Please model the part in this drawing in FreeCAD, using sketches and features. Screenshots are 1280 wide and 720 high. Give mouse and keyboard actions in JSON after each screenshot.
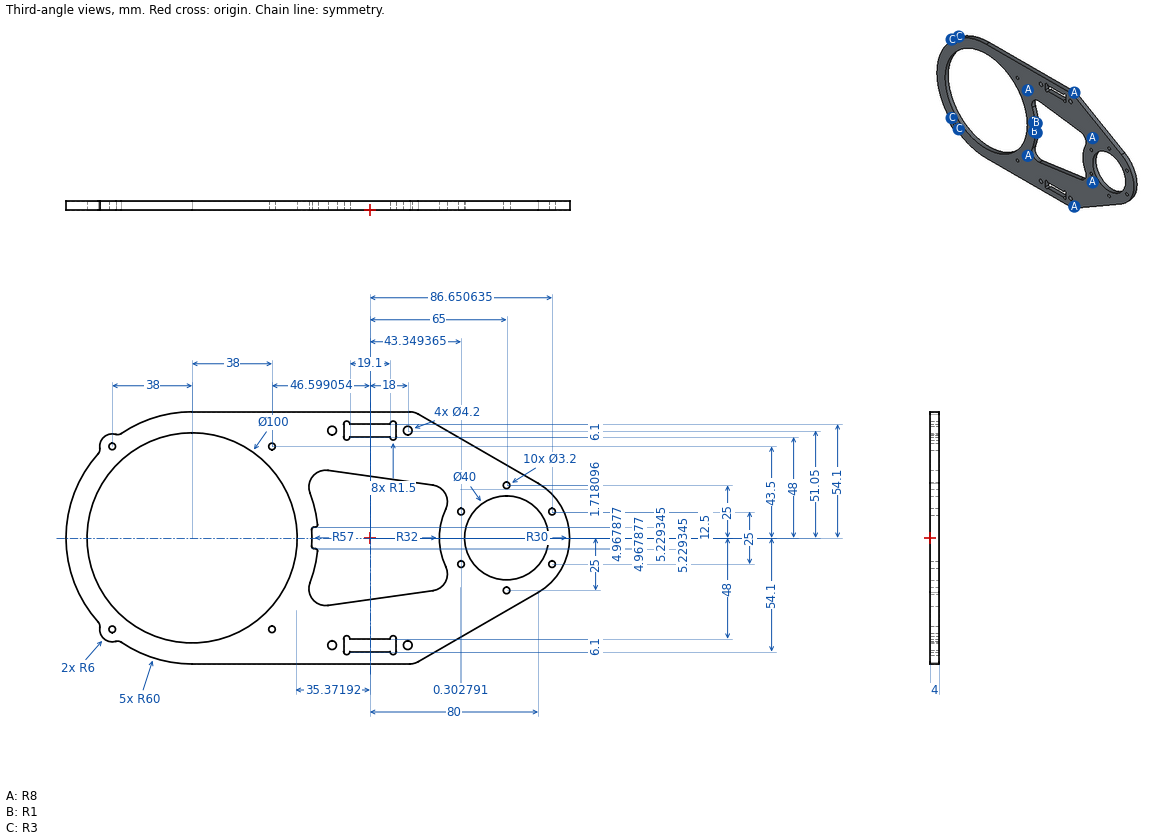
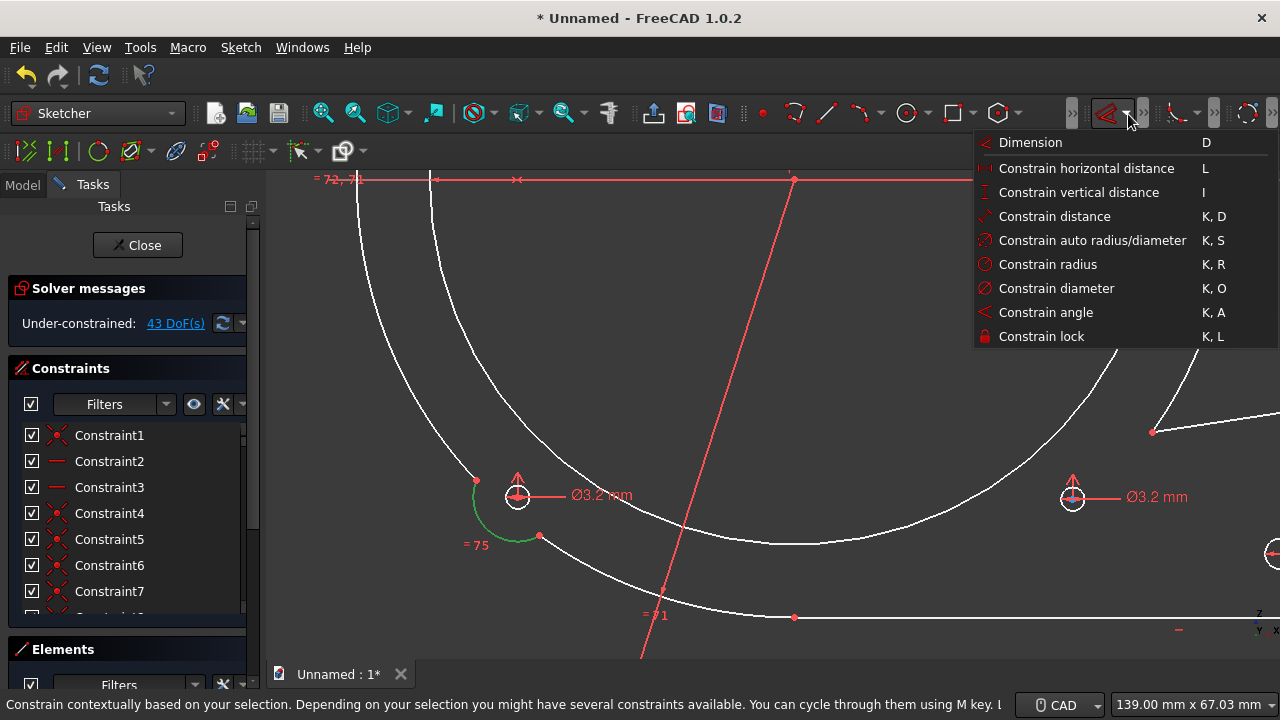
{"action": "left_click", "coordinate": [1126, 264]}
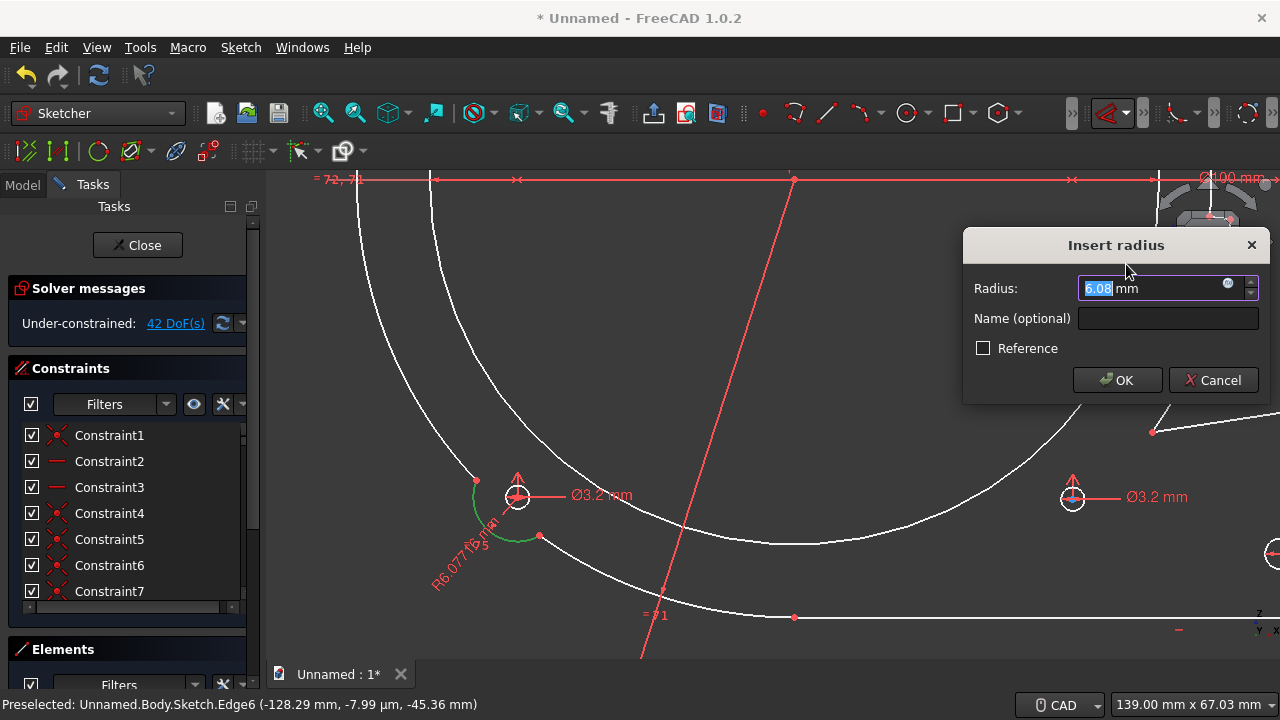
{"action": "type", "text": "6"}
{"action": "key", "text": "Return"}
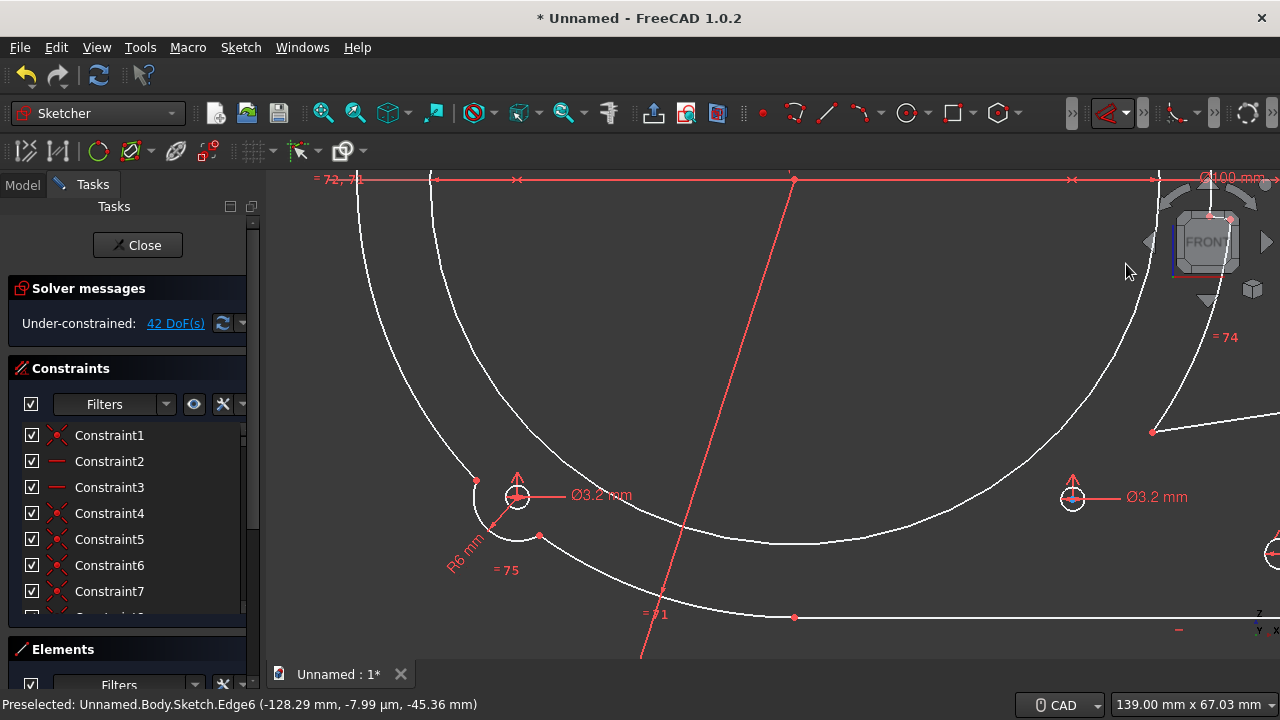
{"action": "scroll", "coordinate": [478, 516], "scroll_direction": "down", "scroll_amount": 6}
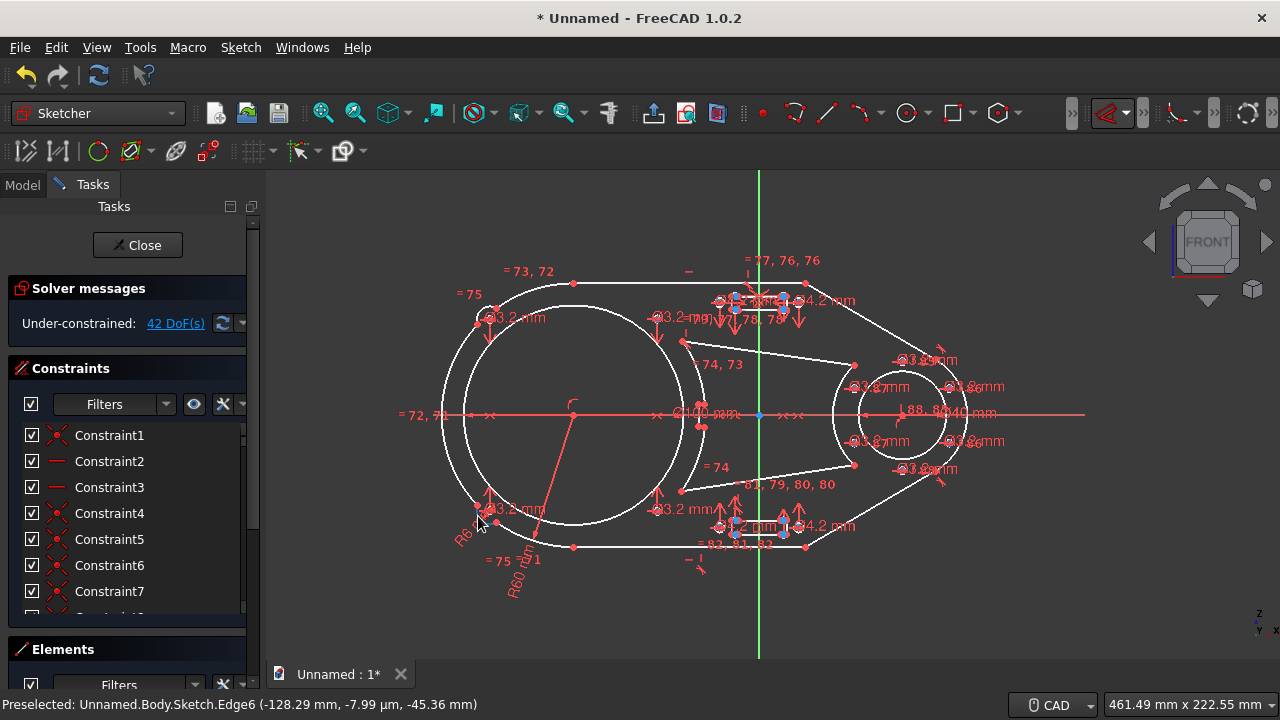
{"action": "scroll", "coordinate": [962, 441], "scroll_direction": "up", "scroll_amount": 3}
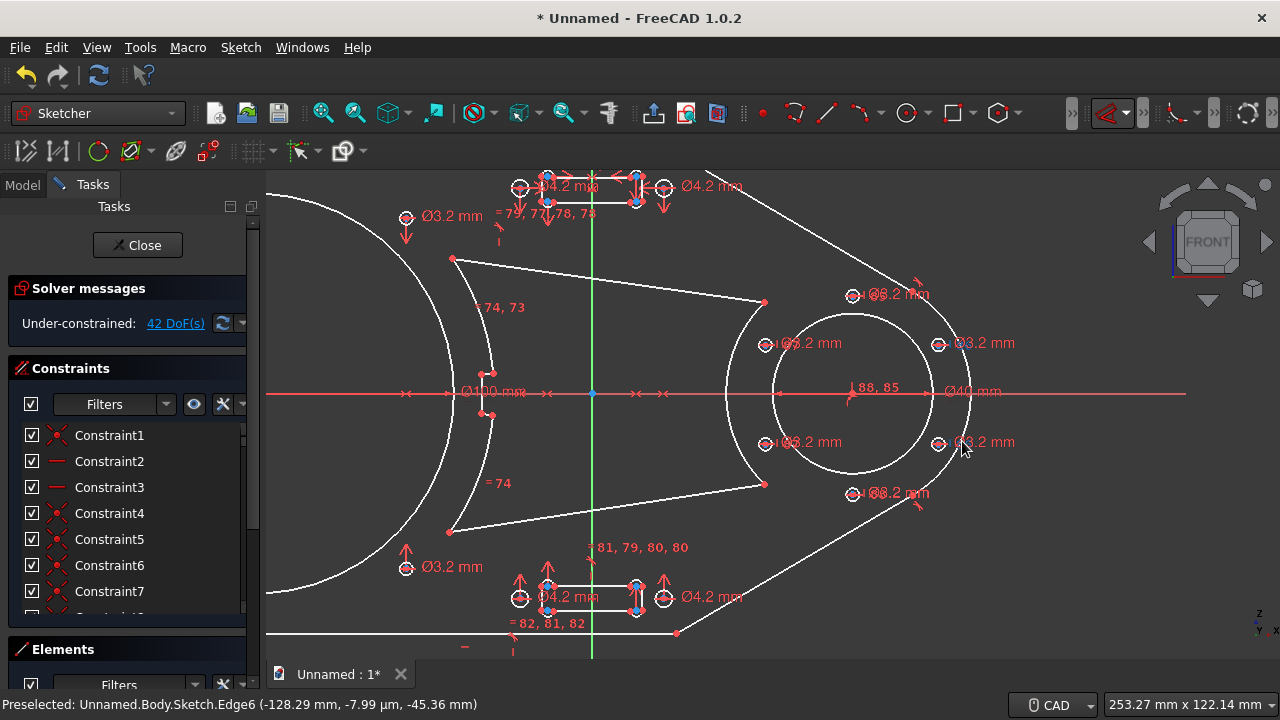
{"action": "left_click", "coordinate": [949, 463]}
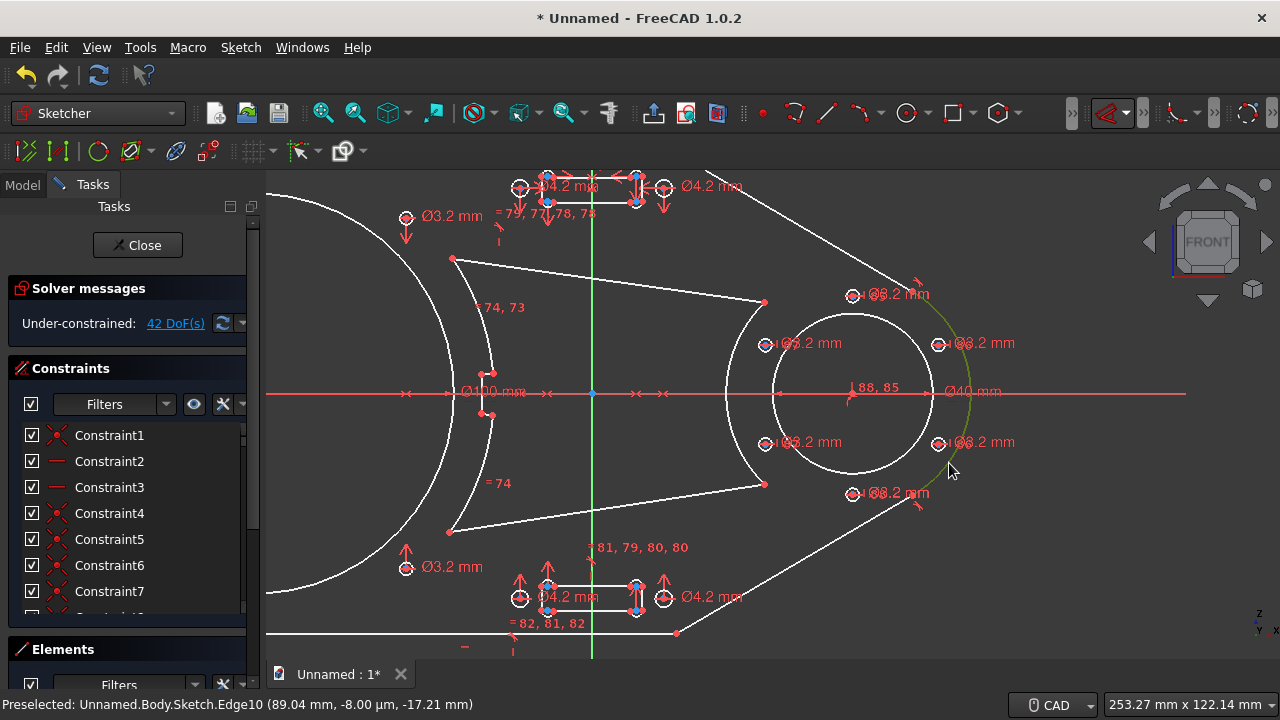
{"action": "key", "text": "k r"}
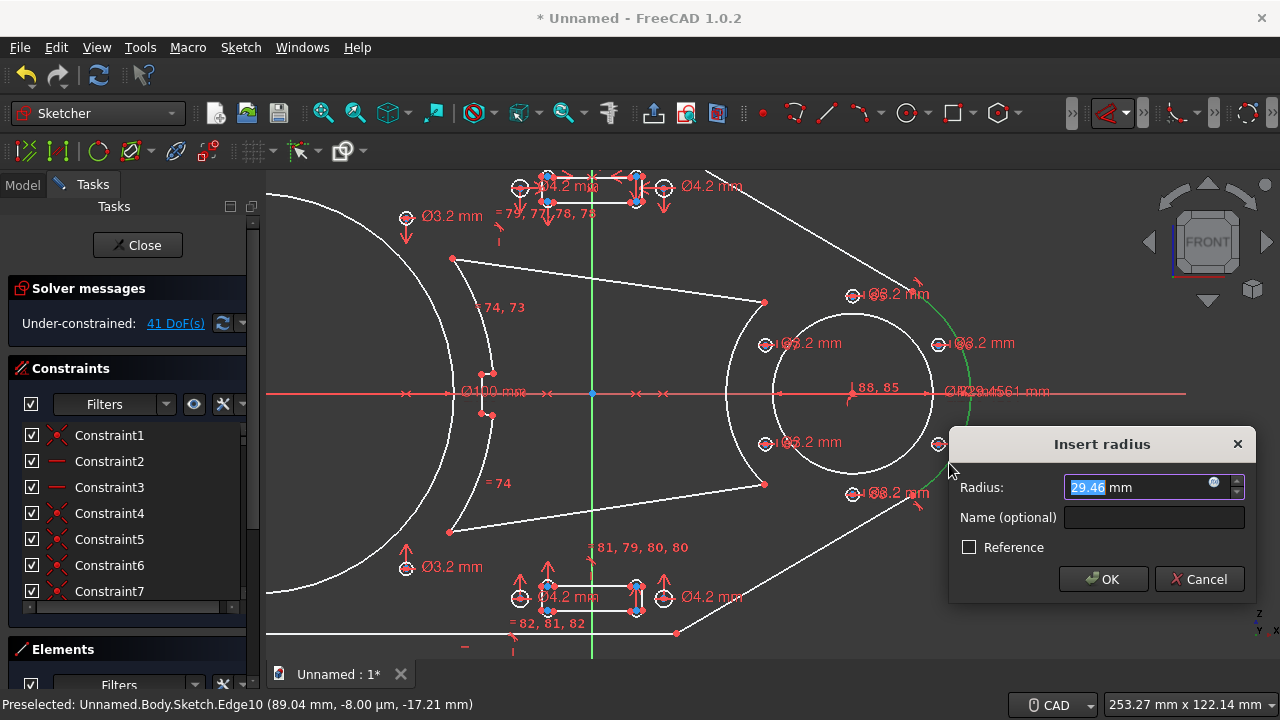
{"action": "type", "text": "30"}
{"action": "key", "text": "Return"}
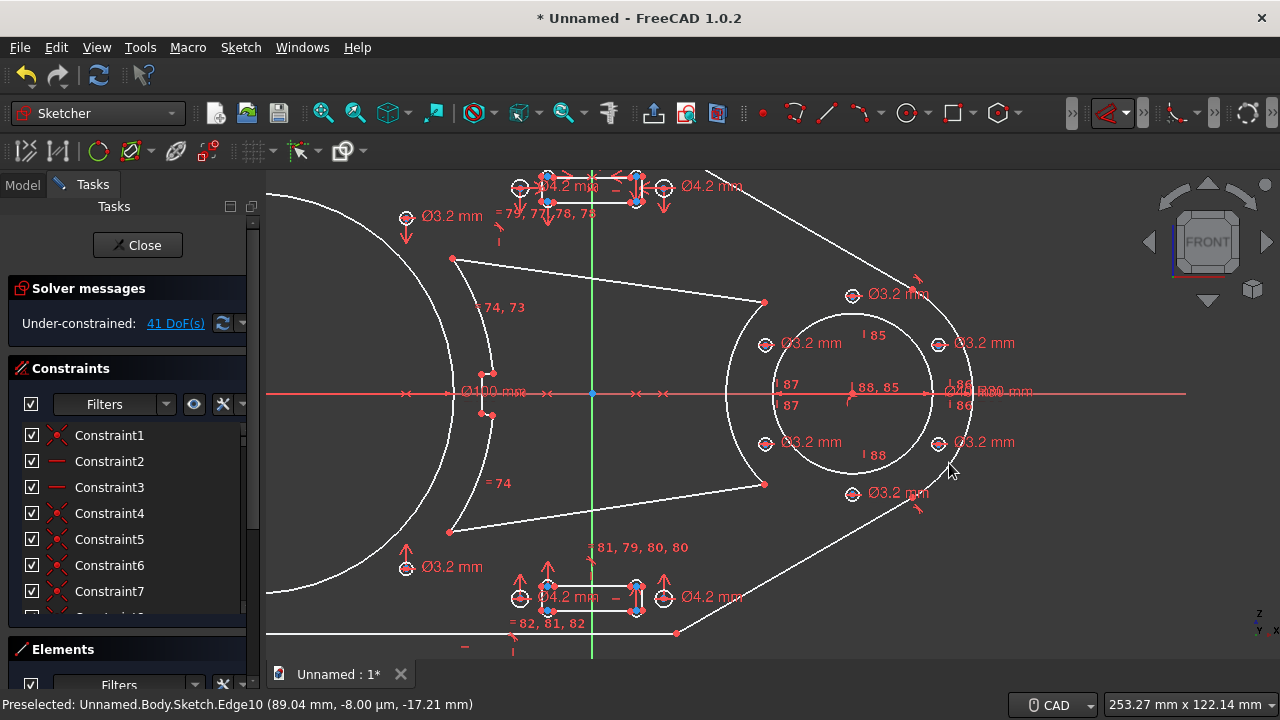
{"action": "scroll", "coordinate": [637, 208], "scroll_direction": "up", "scroll_amount": 10}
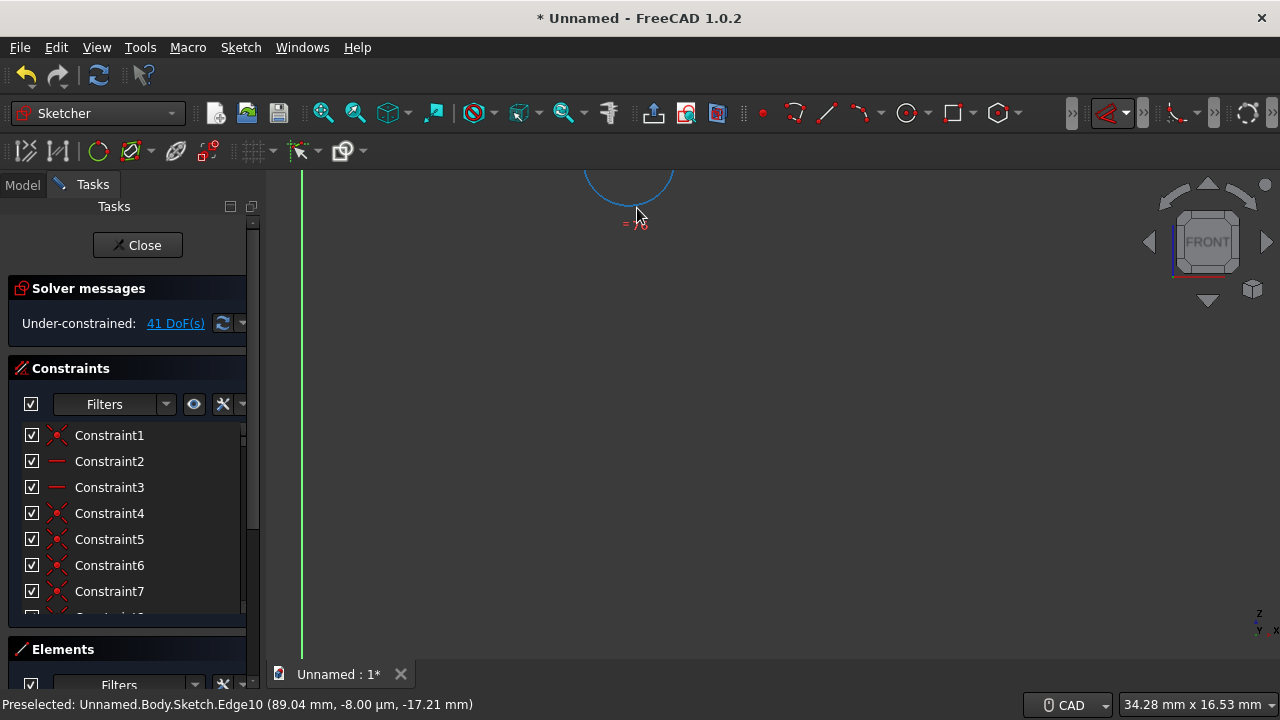
{"action": "left_click", "coordinate": [633, 206]}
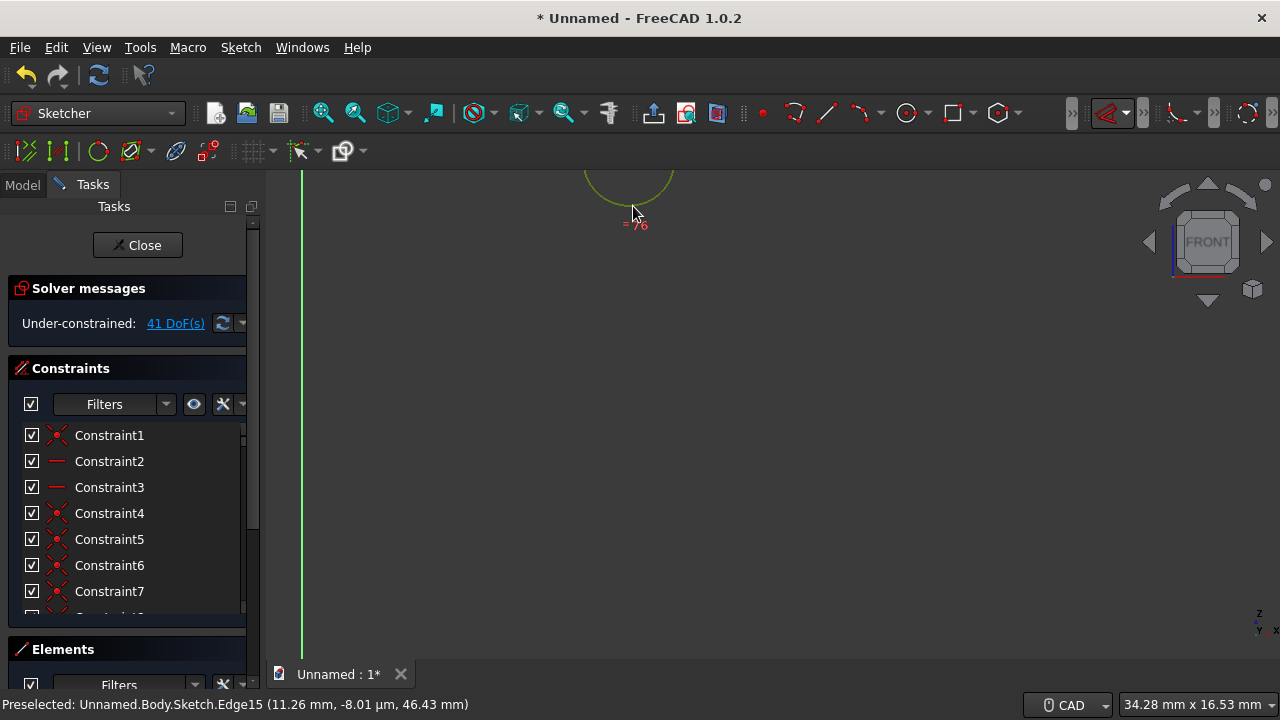
{"action": "left_click", "coordinate": [1128, 114]}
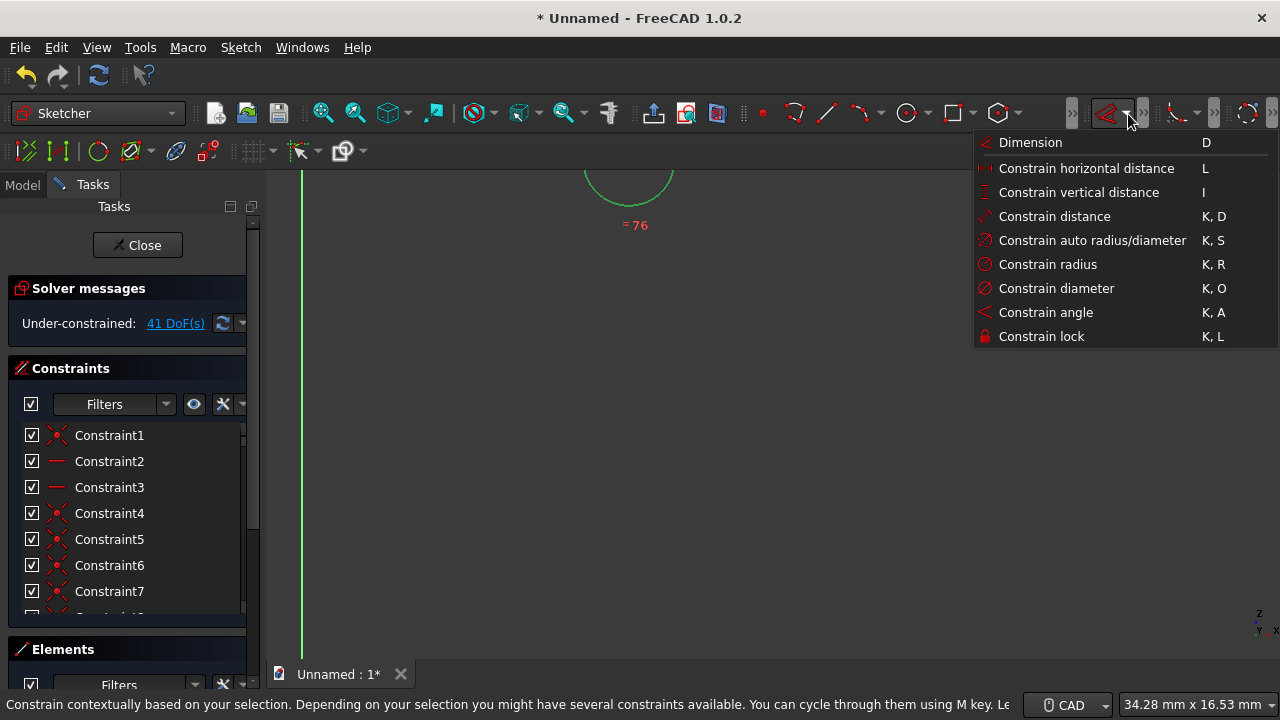
{"action": "left_click", "coordinate": [1126, 264]}